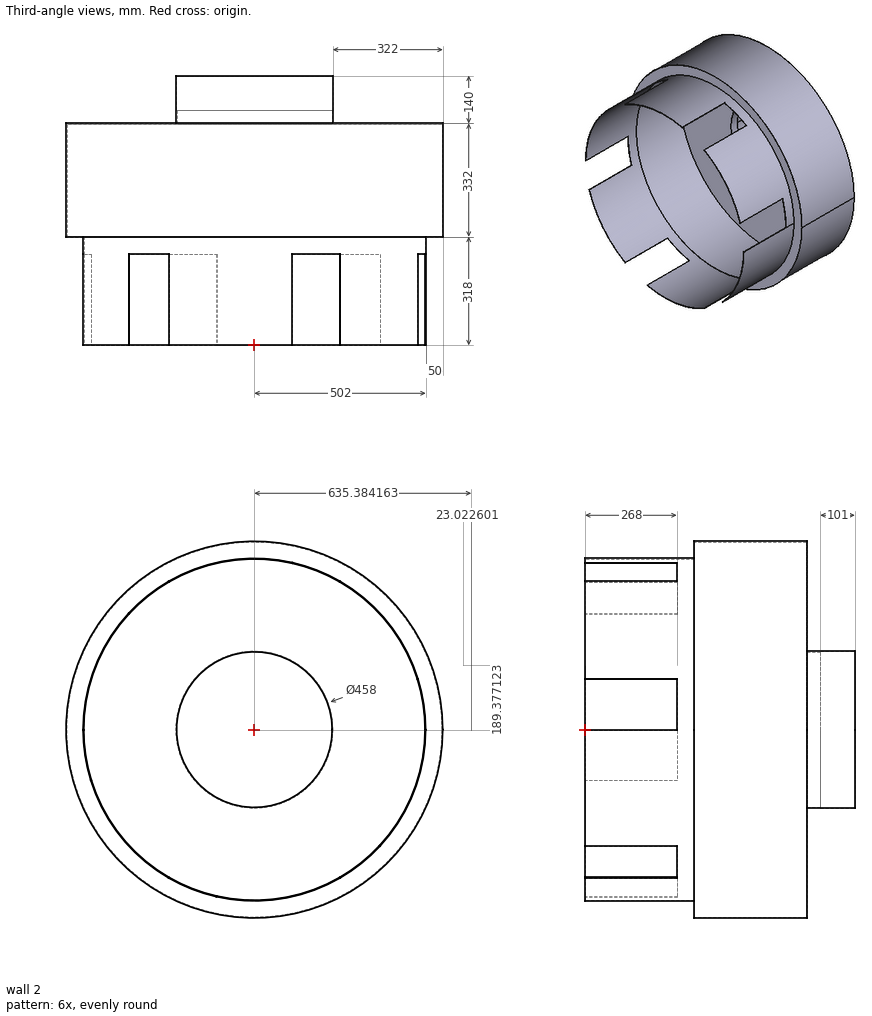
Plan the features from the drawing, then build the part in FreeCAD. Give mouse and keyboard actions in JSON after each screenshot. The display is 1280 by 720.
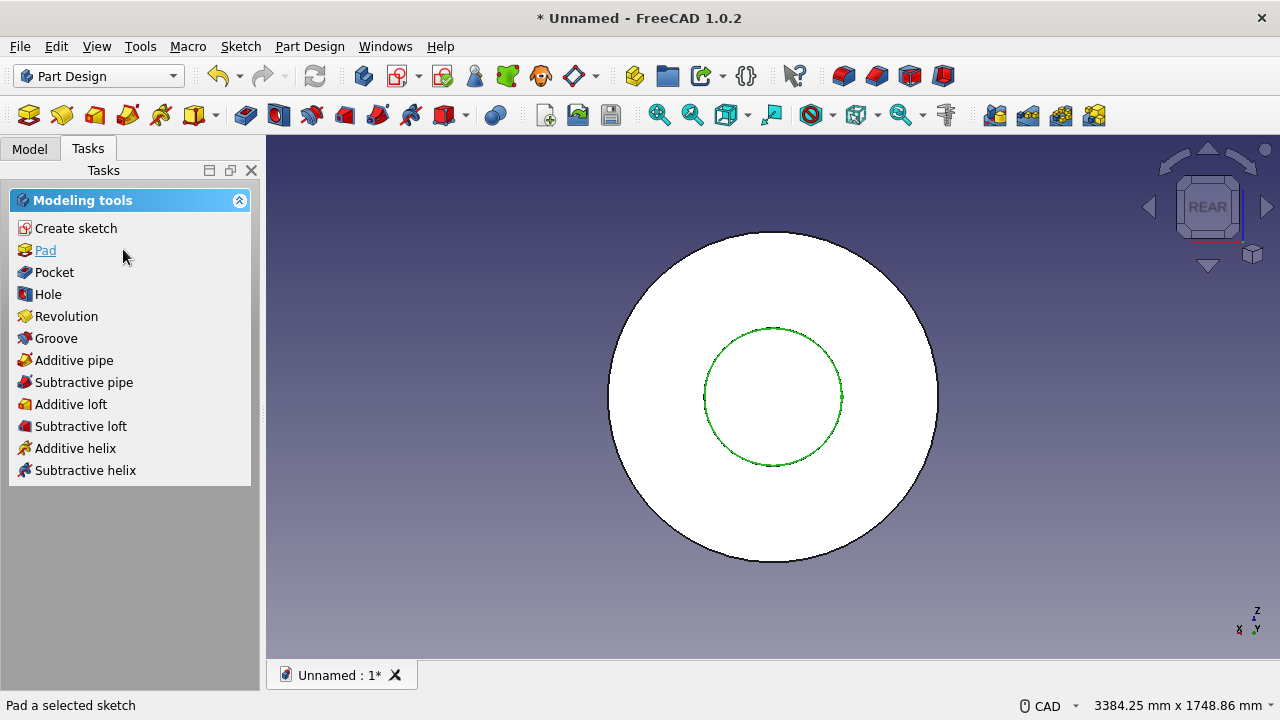
{"action": "left_click", "coordinate": [246, 116]}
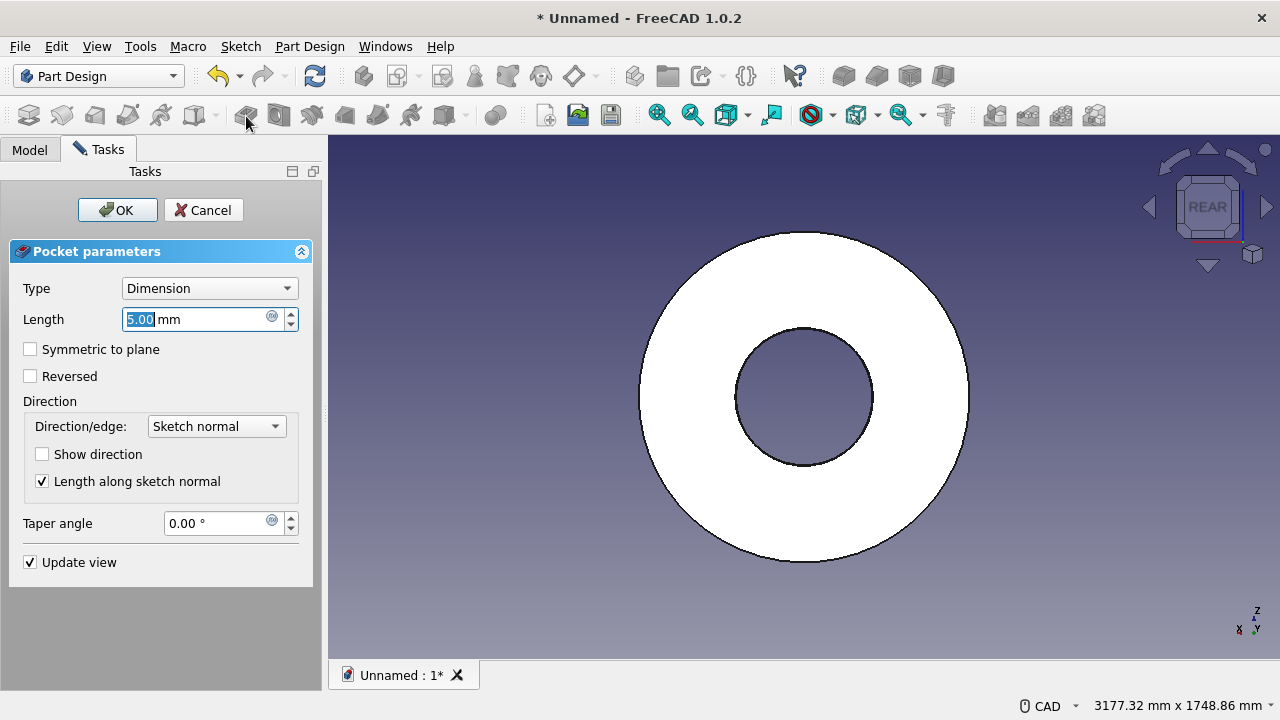
{"action": "type", "text": "101"}
{"action": "key", "text": "Tab"}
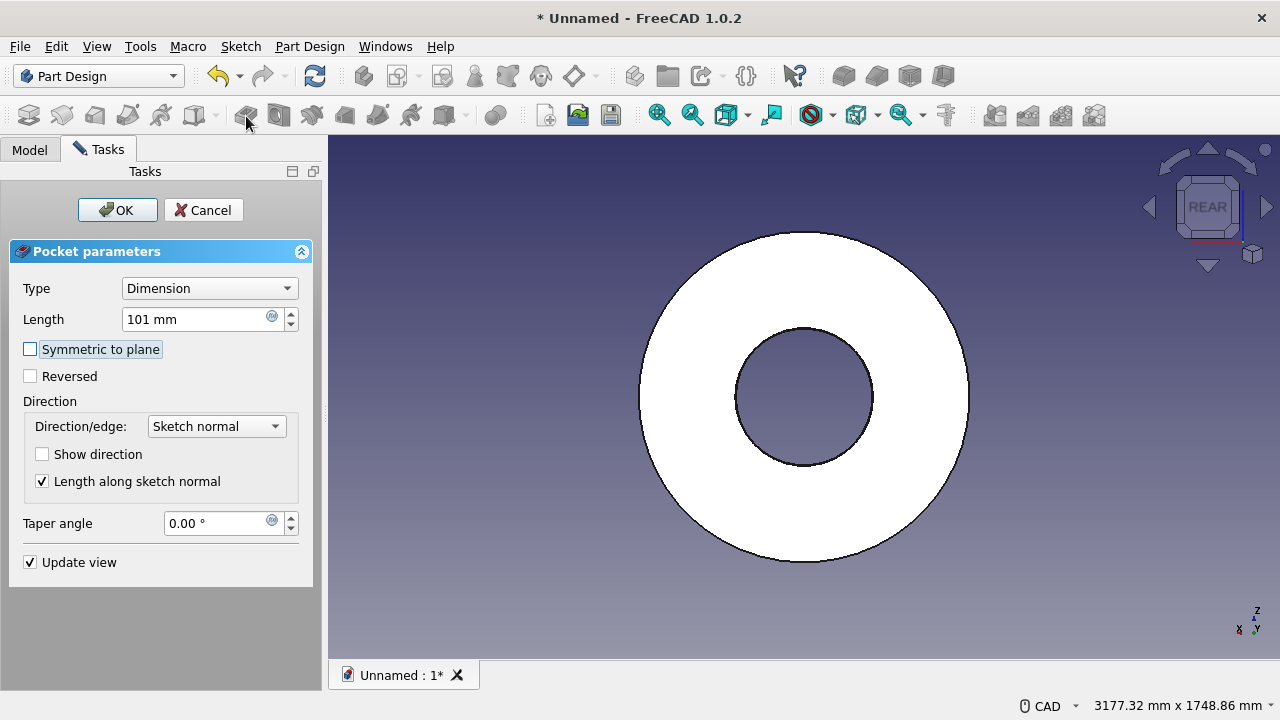
{"action": "left_click", "coordinate": [118, 210]}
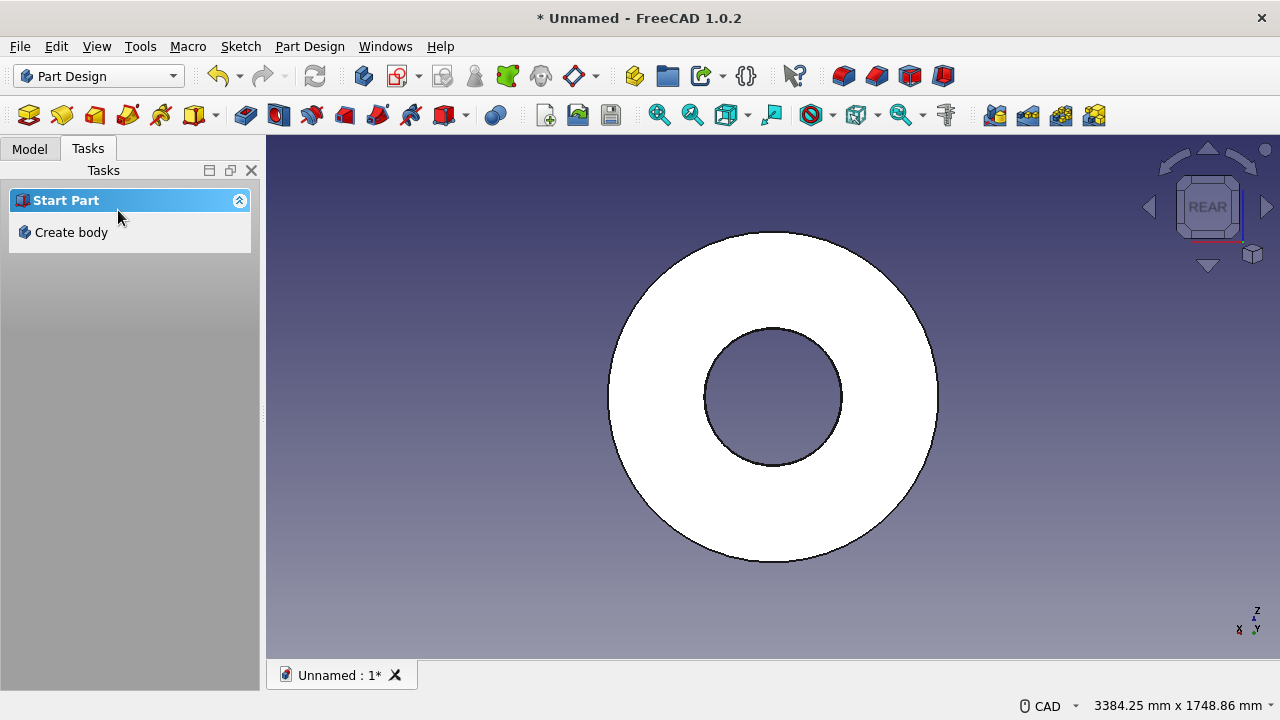
{"action": "key", "text": "0"}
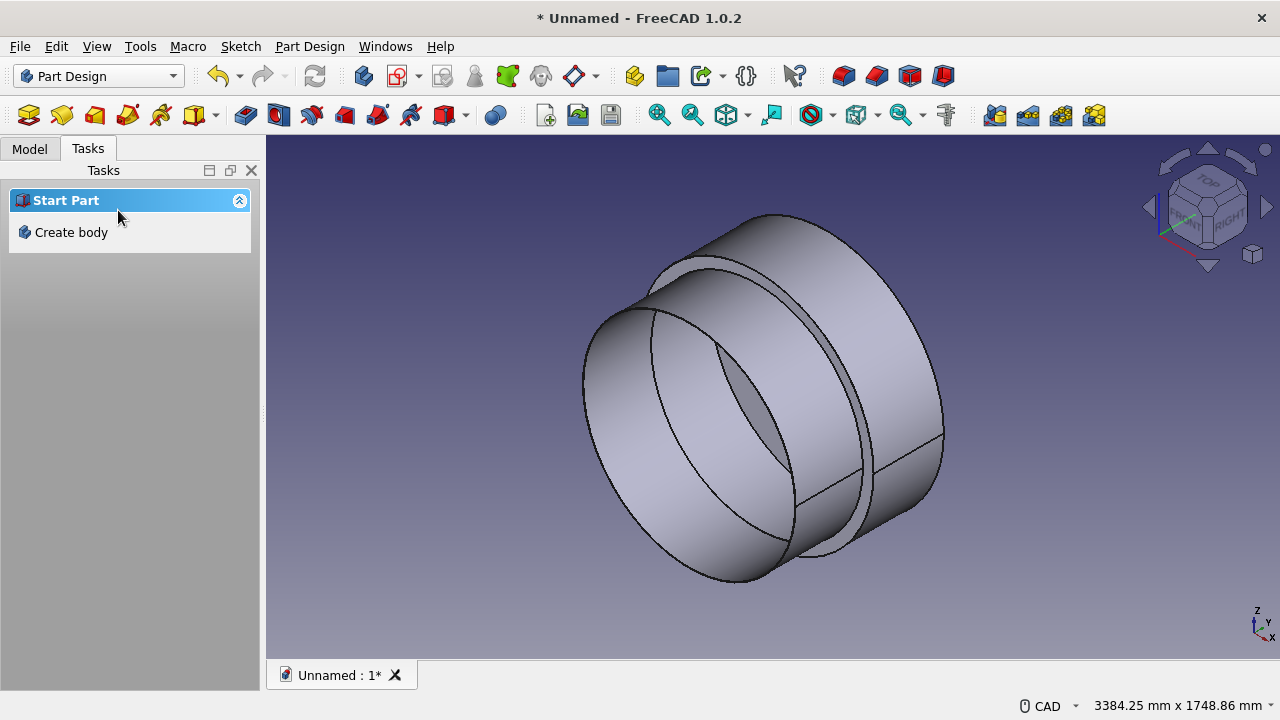
{"action": "scroll", "coordinate": [669, 553], "scroll_direction": "up", "scroll_amount": 15}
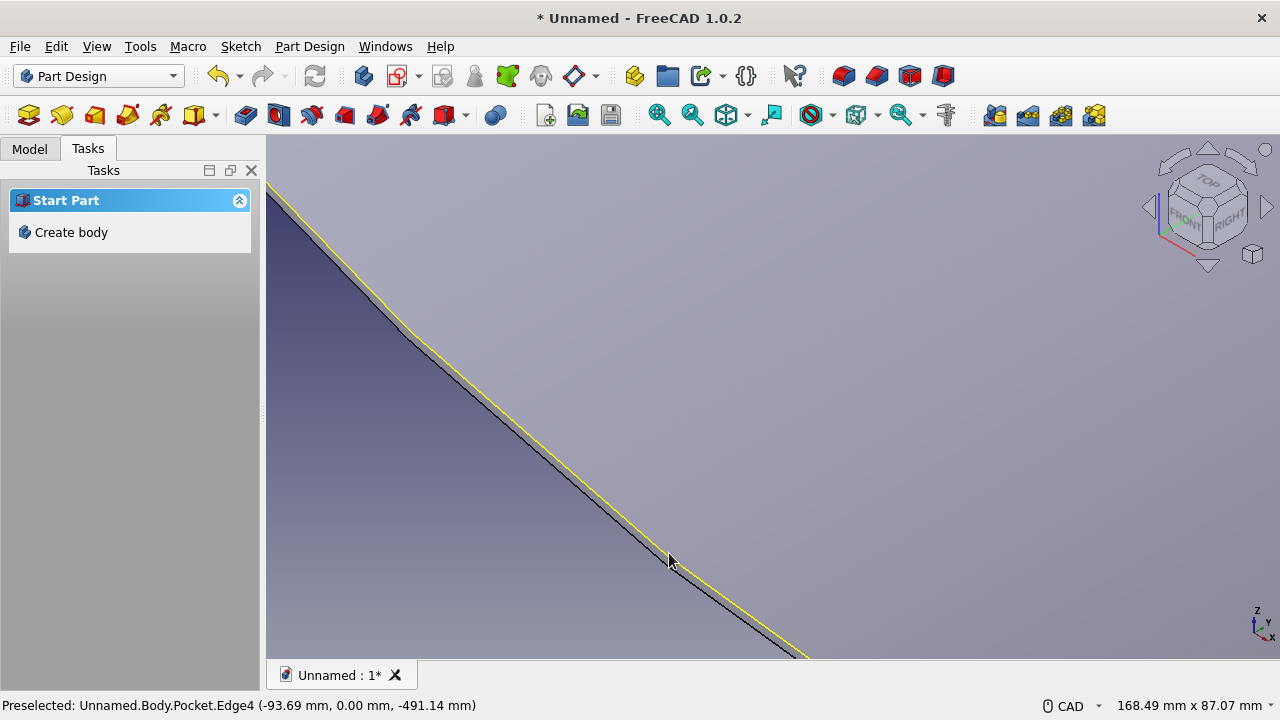
{"action": "scroll", "coordinate": [662, 557], "scroll_direction": "up", "scroll_amount": 5}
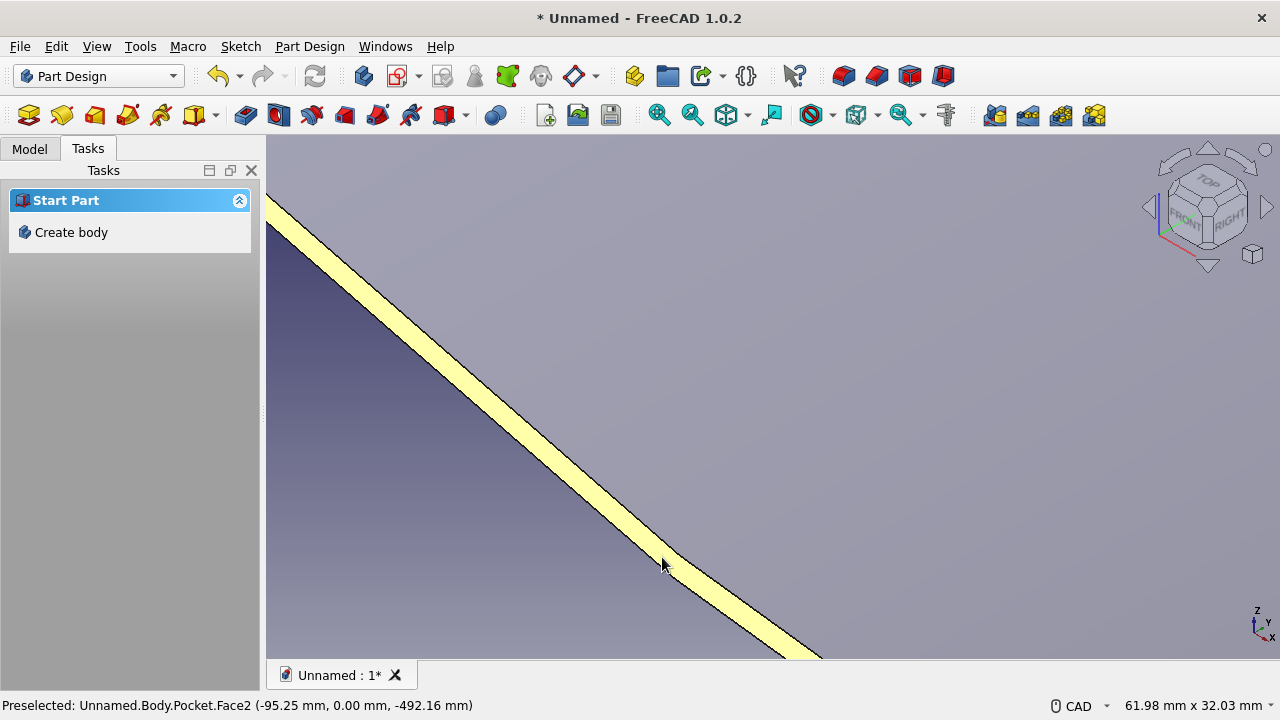
{"action": "left_click", "coordinate": [662, 556]}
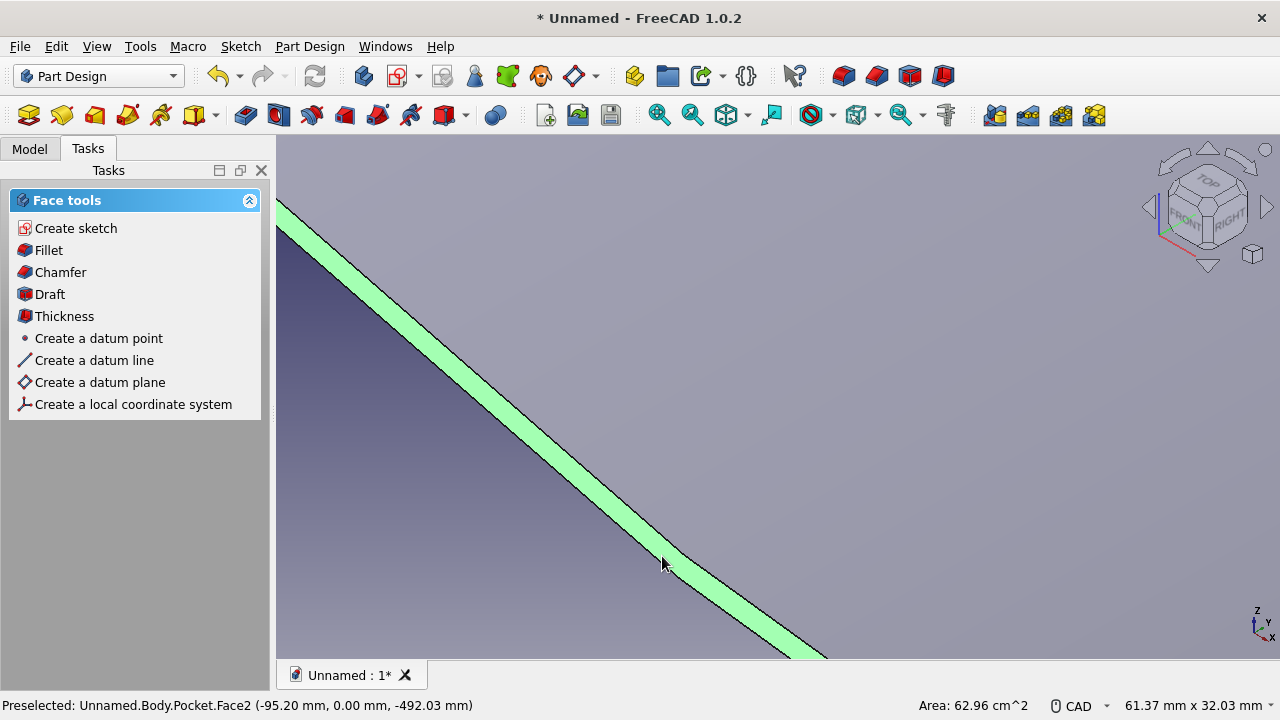
{"action": "left_click", "coordinate": [396, 76]}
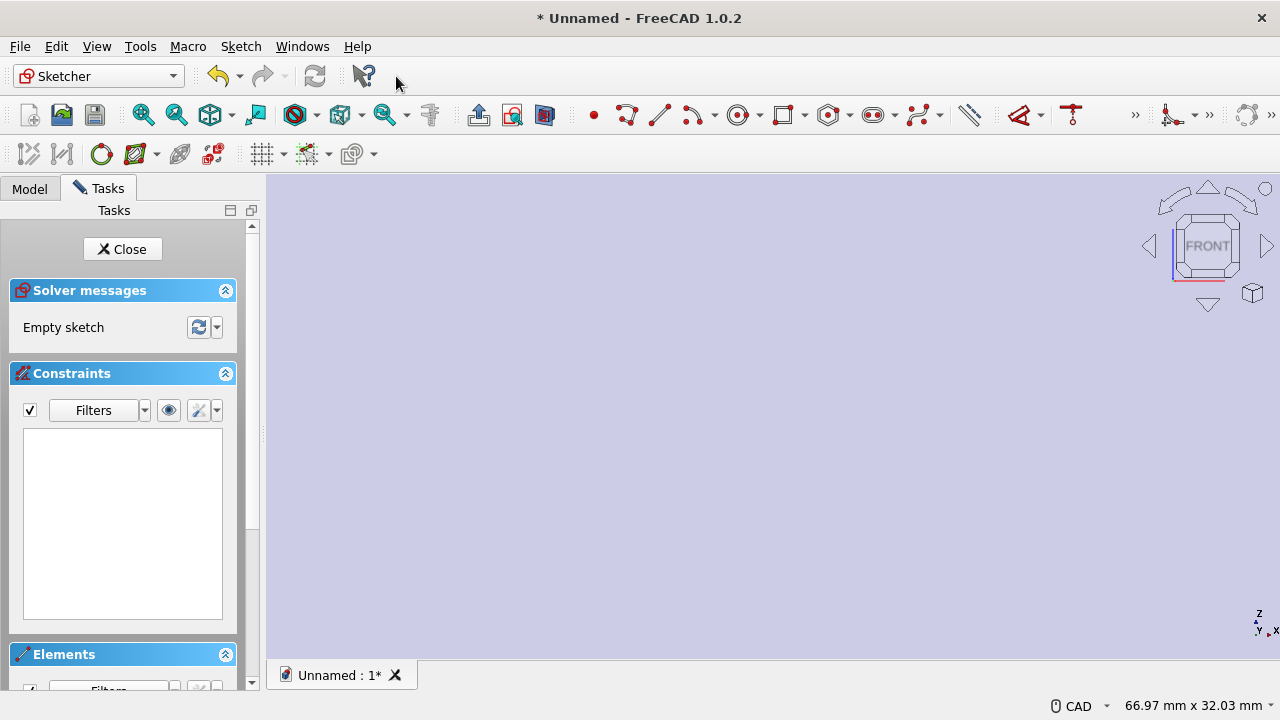
{"action": "scroll", "coordinate": [478, 631], "scroll_direction": "down", "scroll_amount": 16}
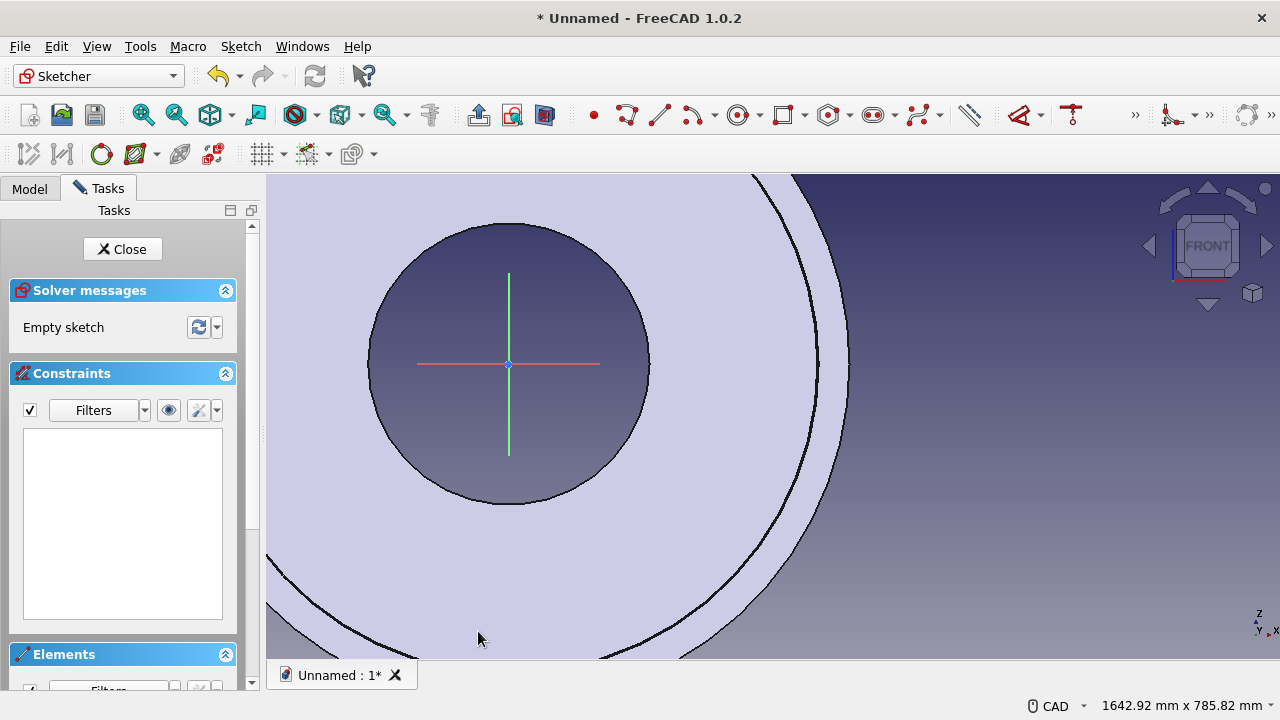
{"action": "scroll", "coordinate": [706, 202], "scroll_direction": "up", "scroll_amount": 2}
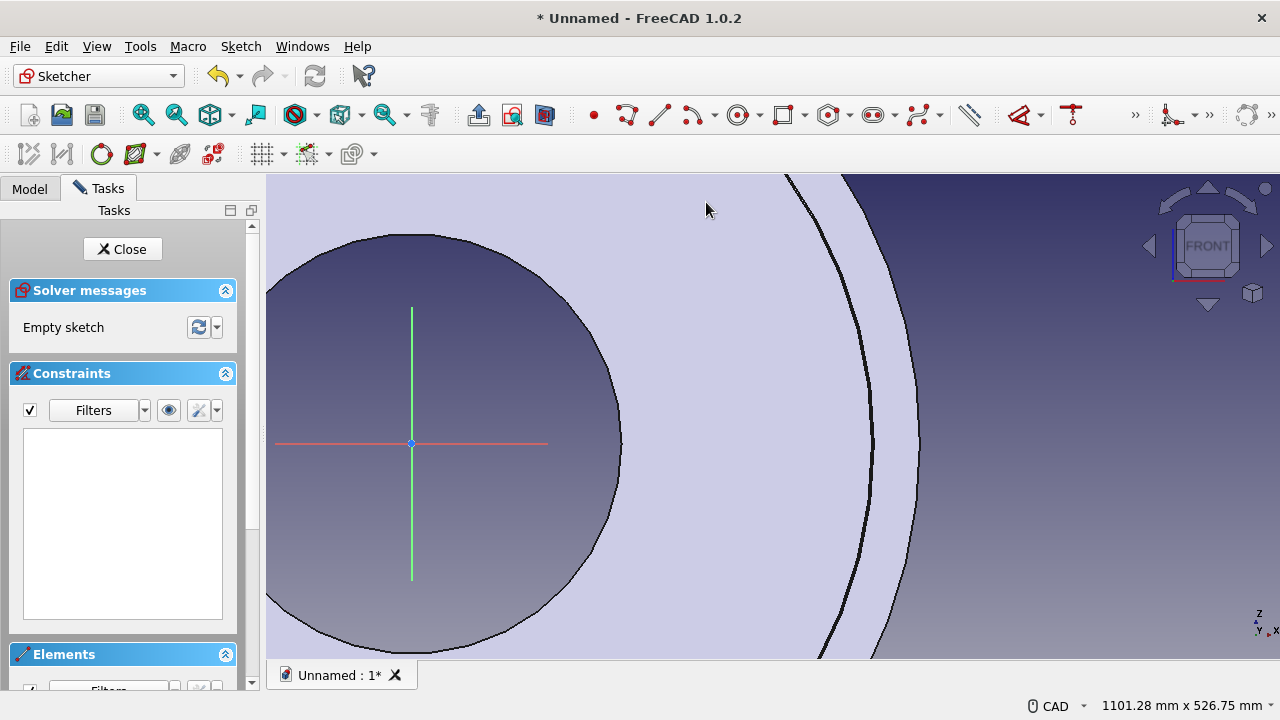
{"action": "left_click", "coordinate": [627, 116]}